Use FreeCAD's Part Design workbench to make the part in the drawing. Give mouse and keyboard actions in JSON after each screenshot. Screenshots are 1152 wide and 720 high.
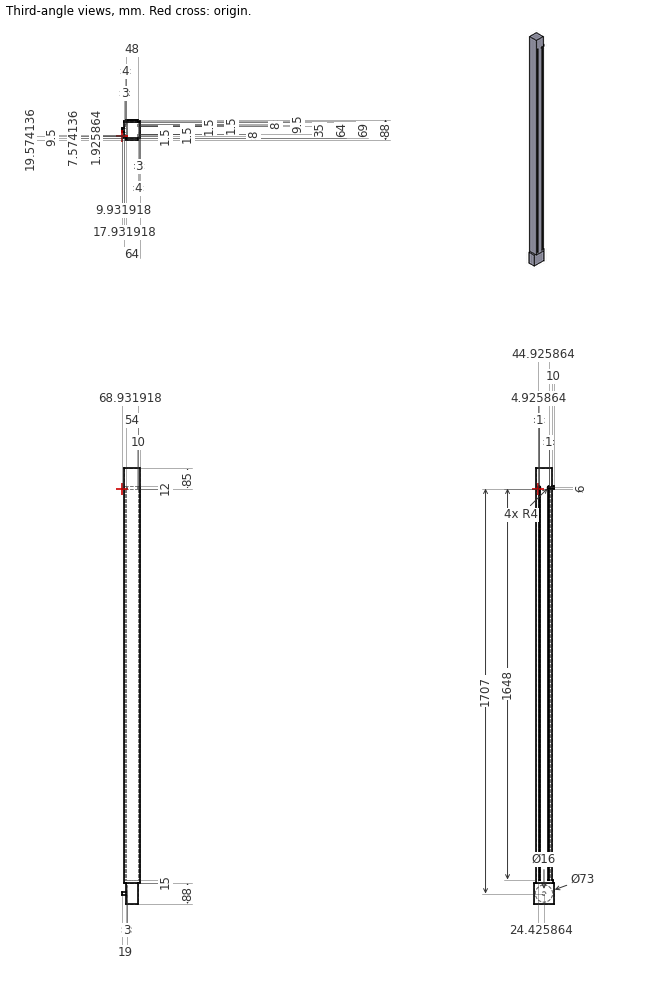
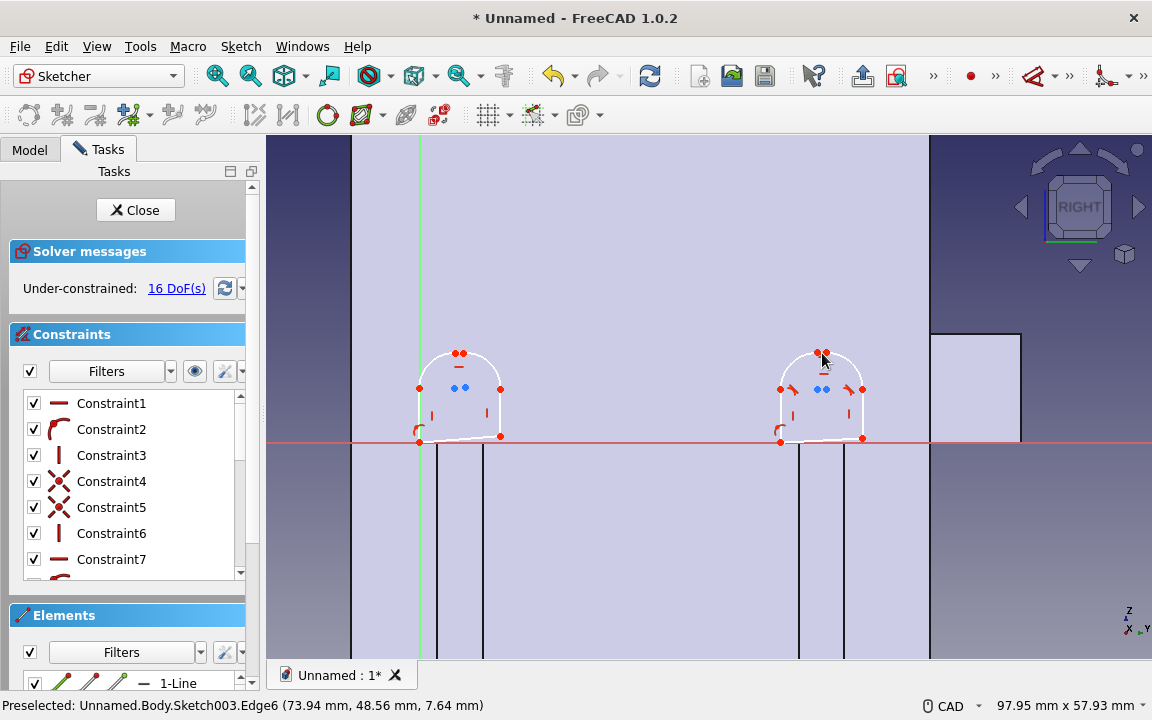
{"action": "scroll", "coordinate": [461, 353], "scroll_direction": "up", "scroll_amount": 8}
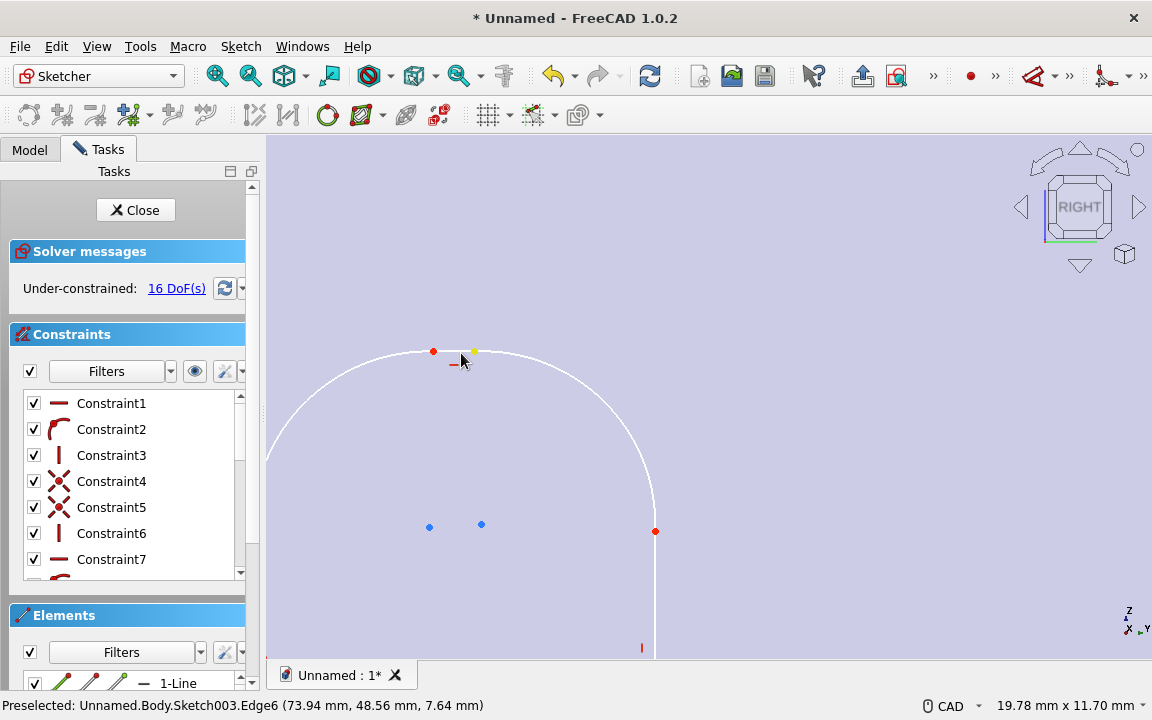
{"action": "left_click", "coordinate": [458, 351]}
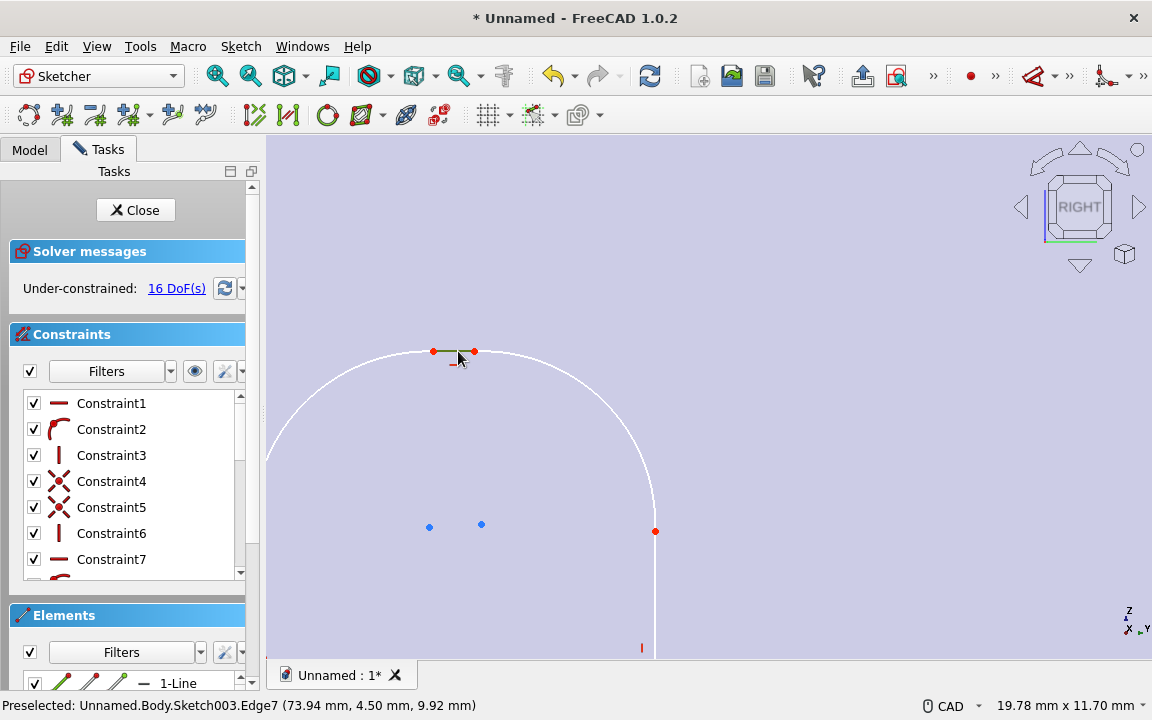
{"action": "scroll", "coordinate": [461, 353], "scroll_direction": "down", "scroll_amount": 8}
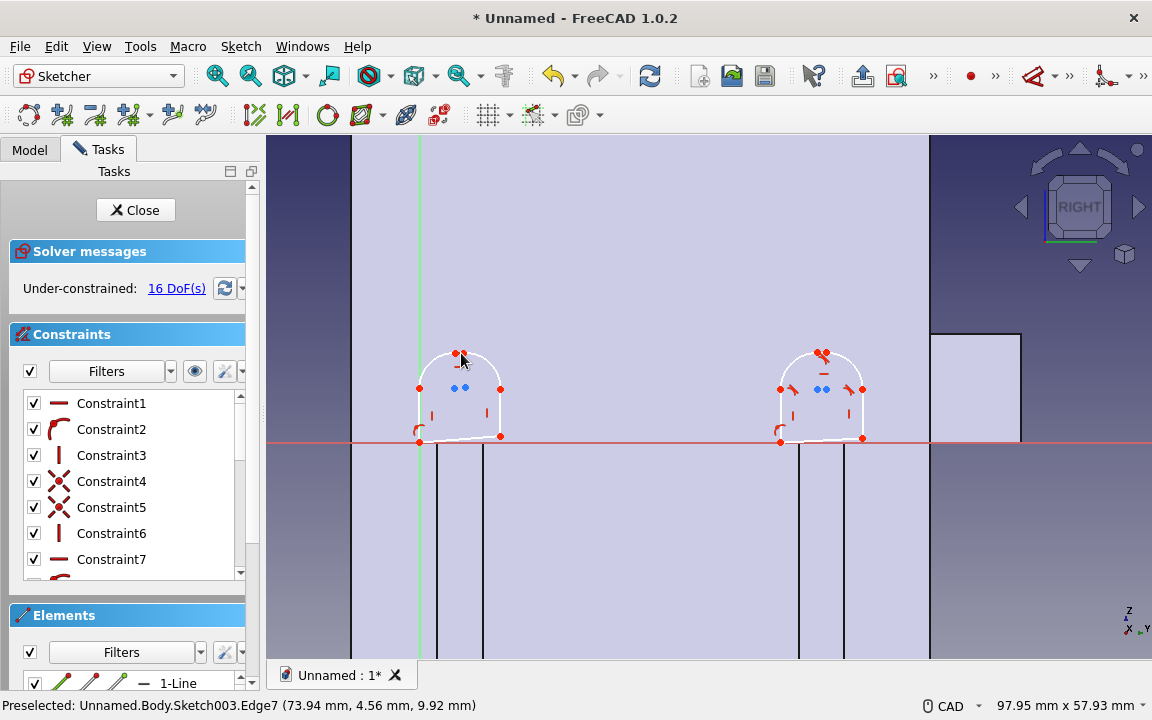
{"action": "left_click", "coordinate": [439, 357]}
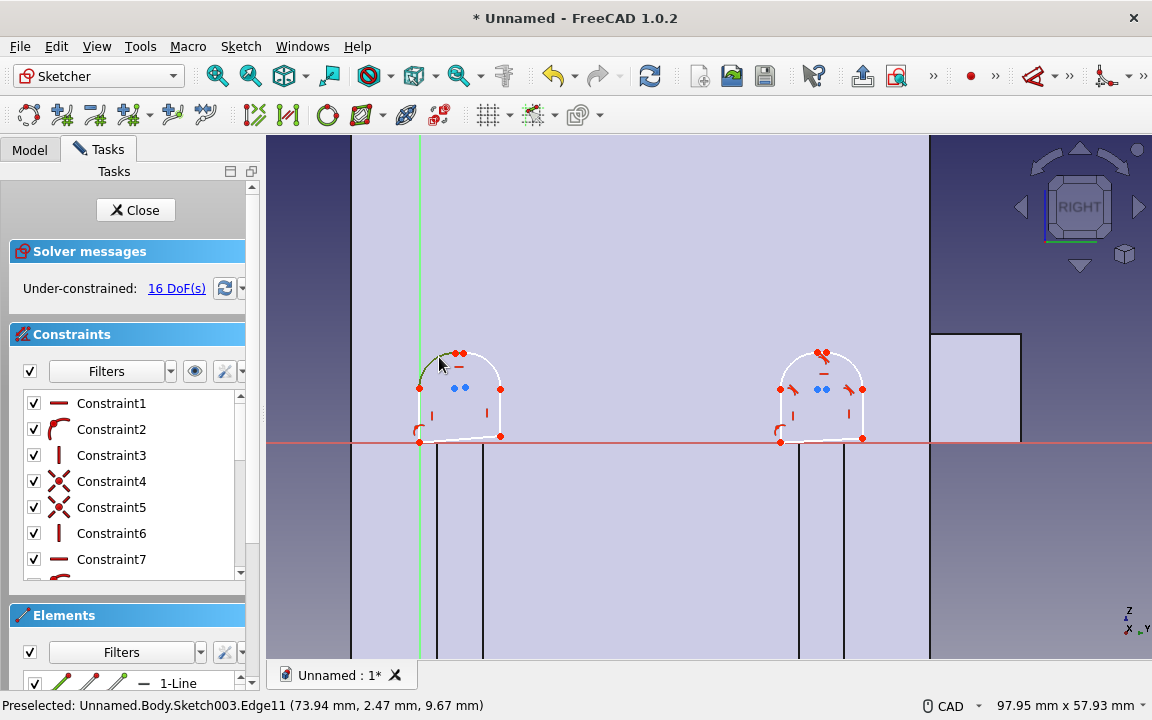
{"action": "key", "text": "t"}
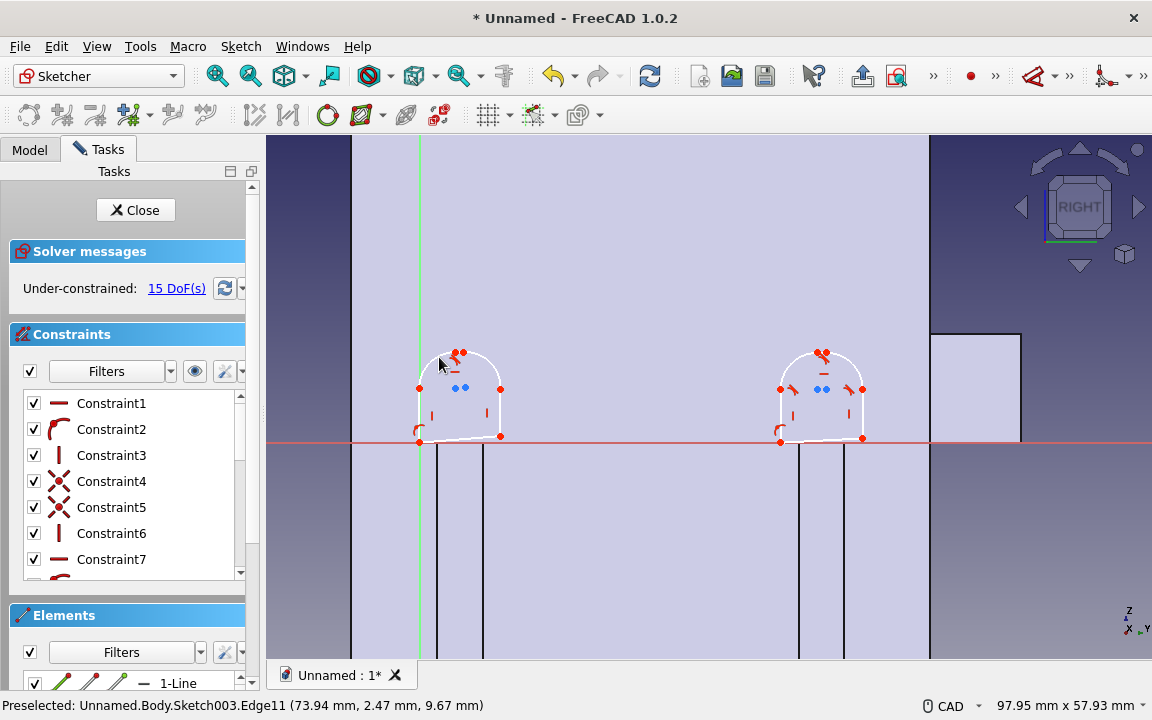
{"action": "scroll", "coordinate": [460, 352], "scroll_direction": "up", "scroll_amount": 6}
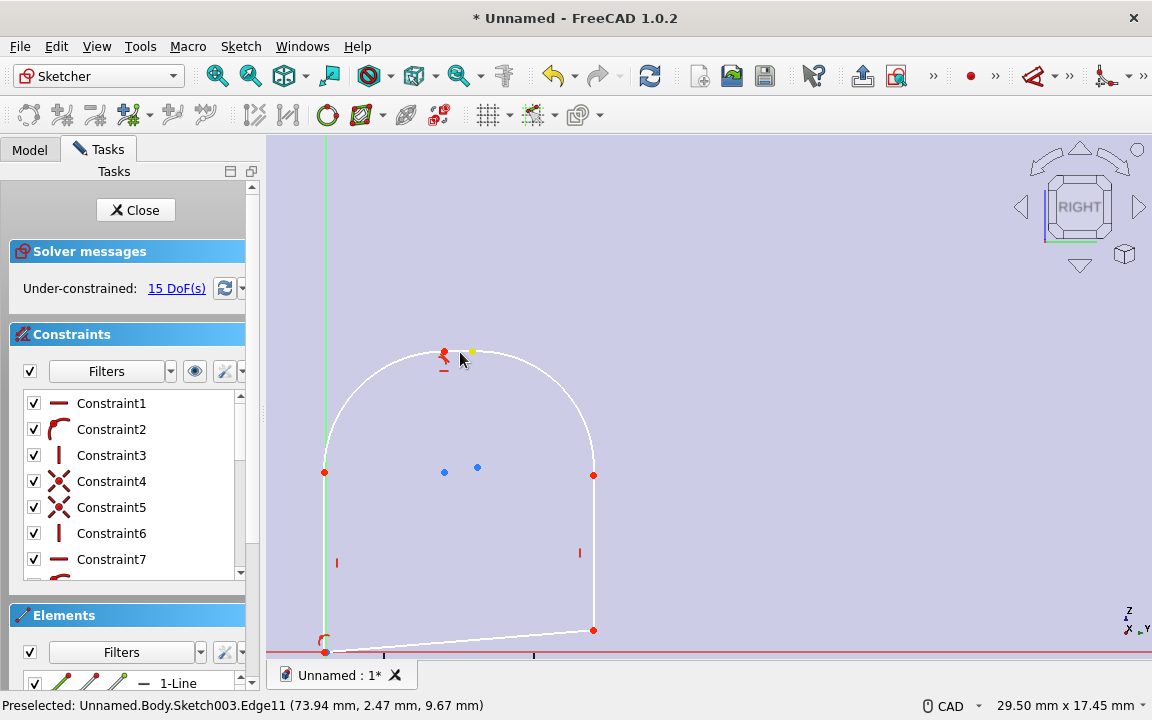
{"action": "left_click", "coordinate": [459, 351]}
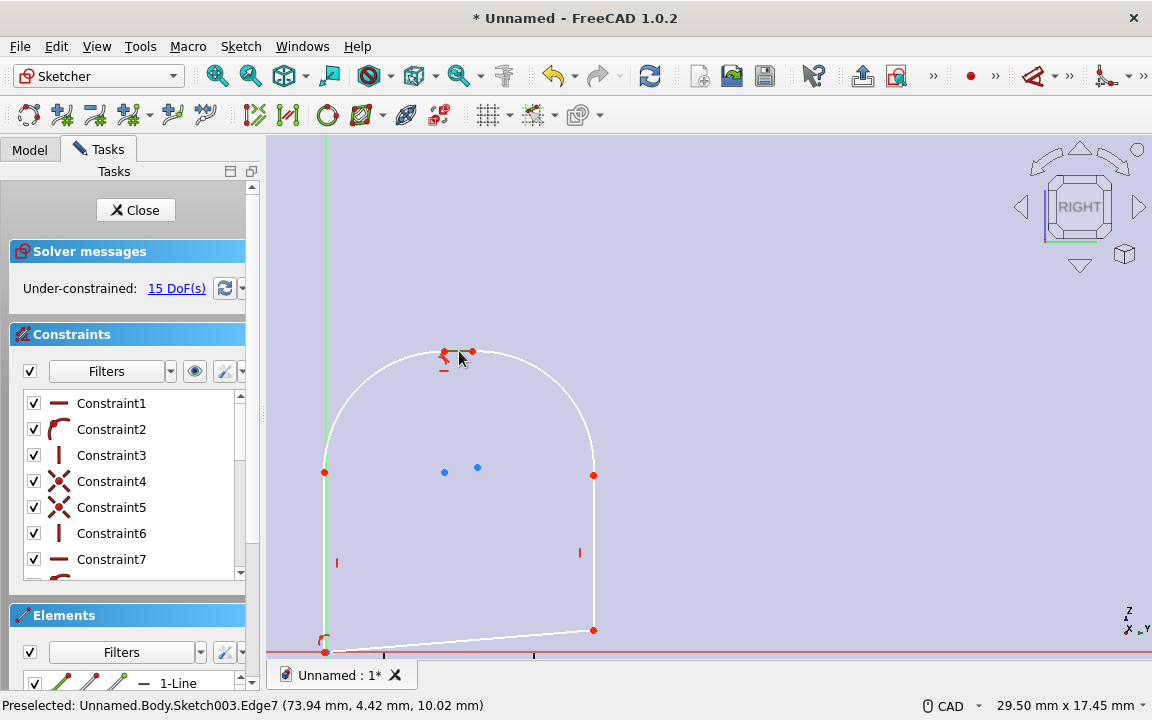
{"action": "left_click", "coordinate": [583, 418]}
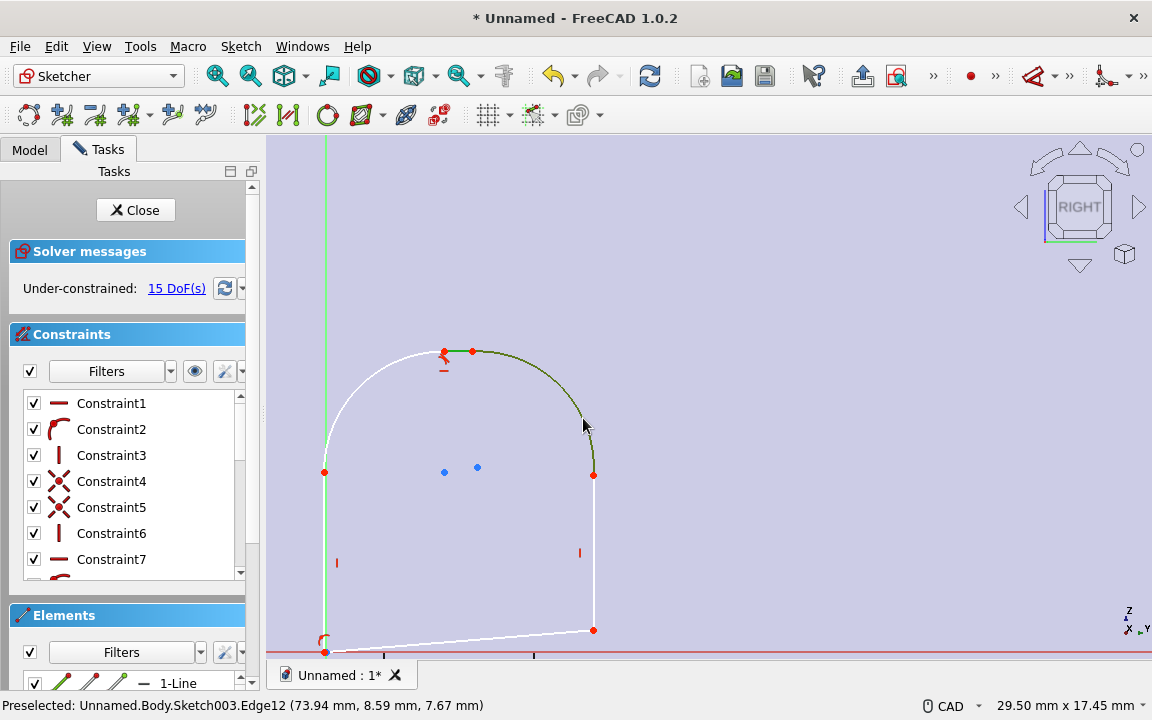
{"action": "key", "text": "t"}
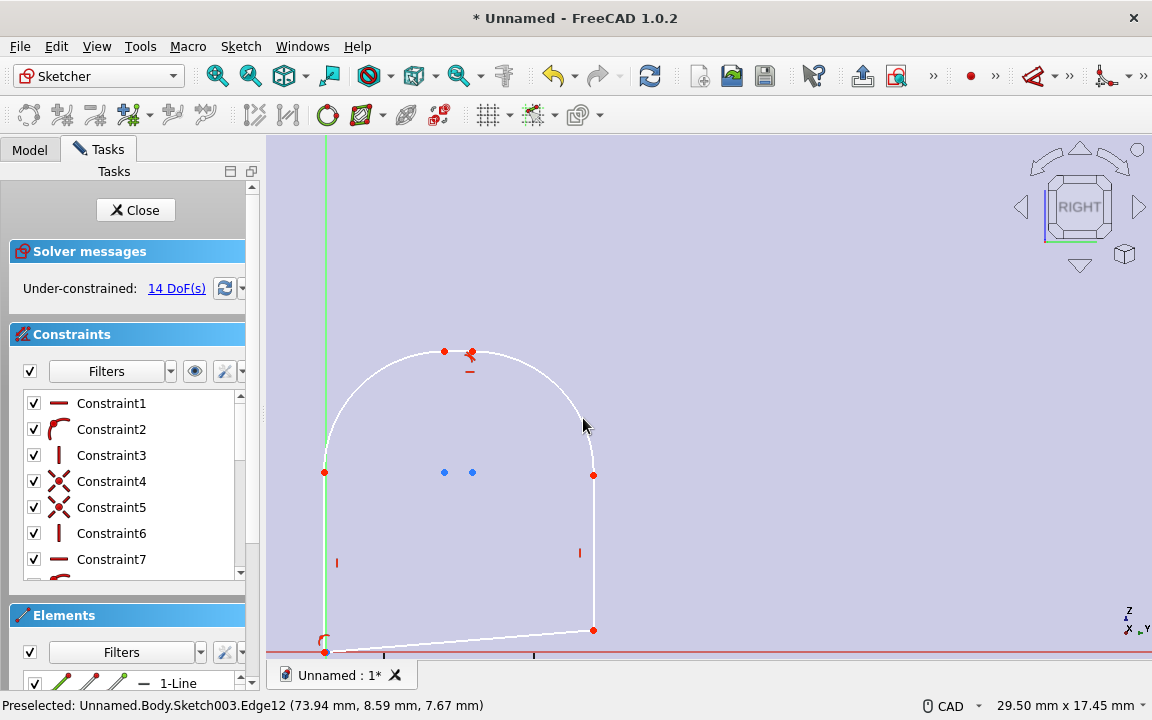
{"action": "left_click", "coordinate": [324, 526]}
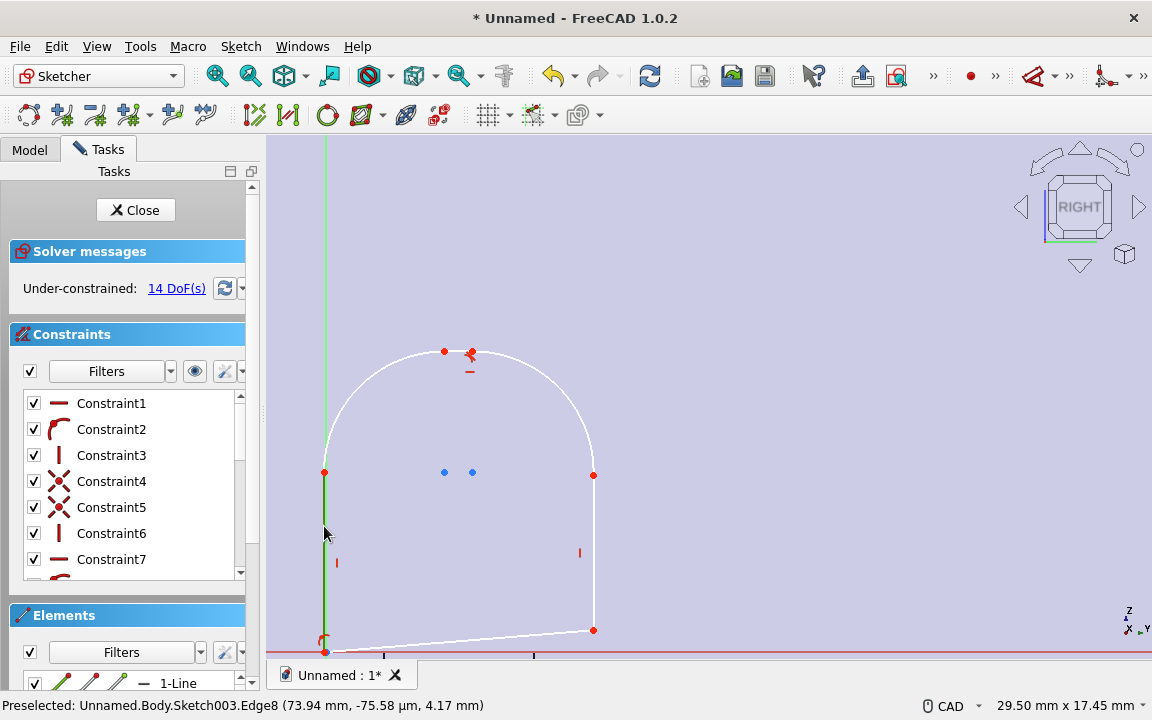
{"action": "left_click", "coordinate": [390, 365]}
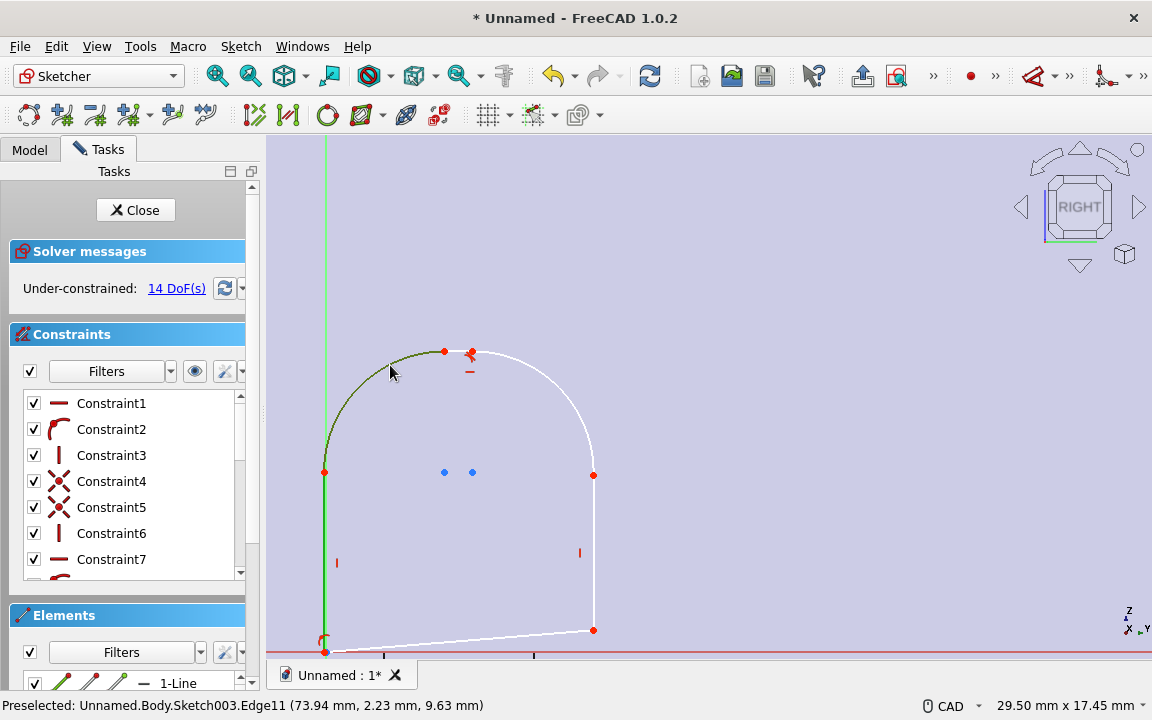
{"action": "key", "text": "t"}